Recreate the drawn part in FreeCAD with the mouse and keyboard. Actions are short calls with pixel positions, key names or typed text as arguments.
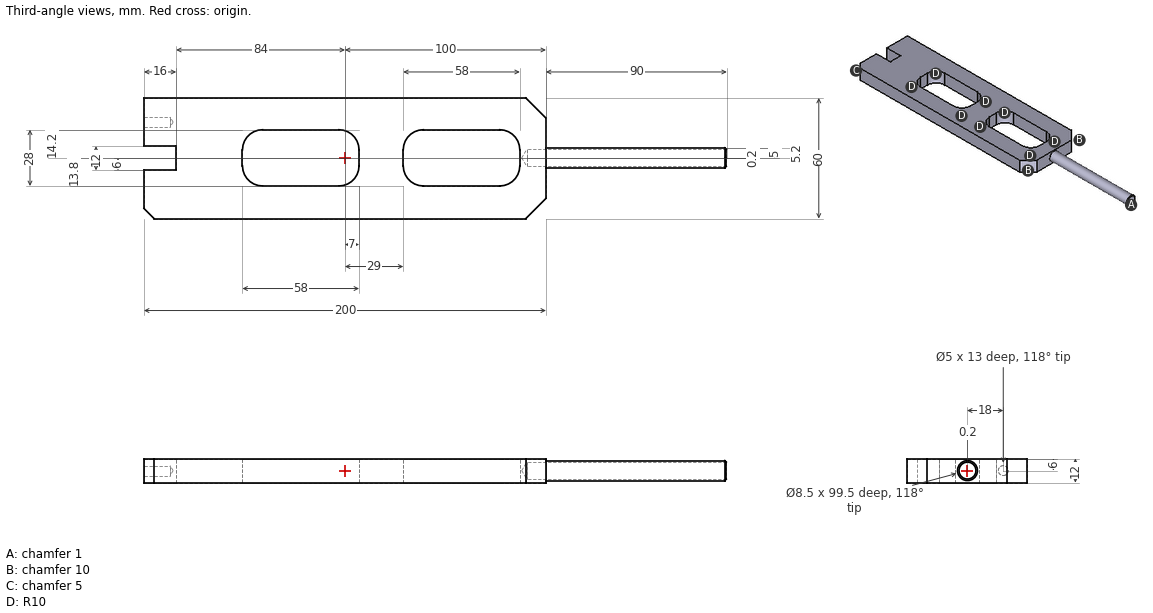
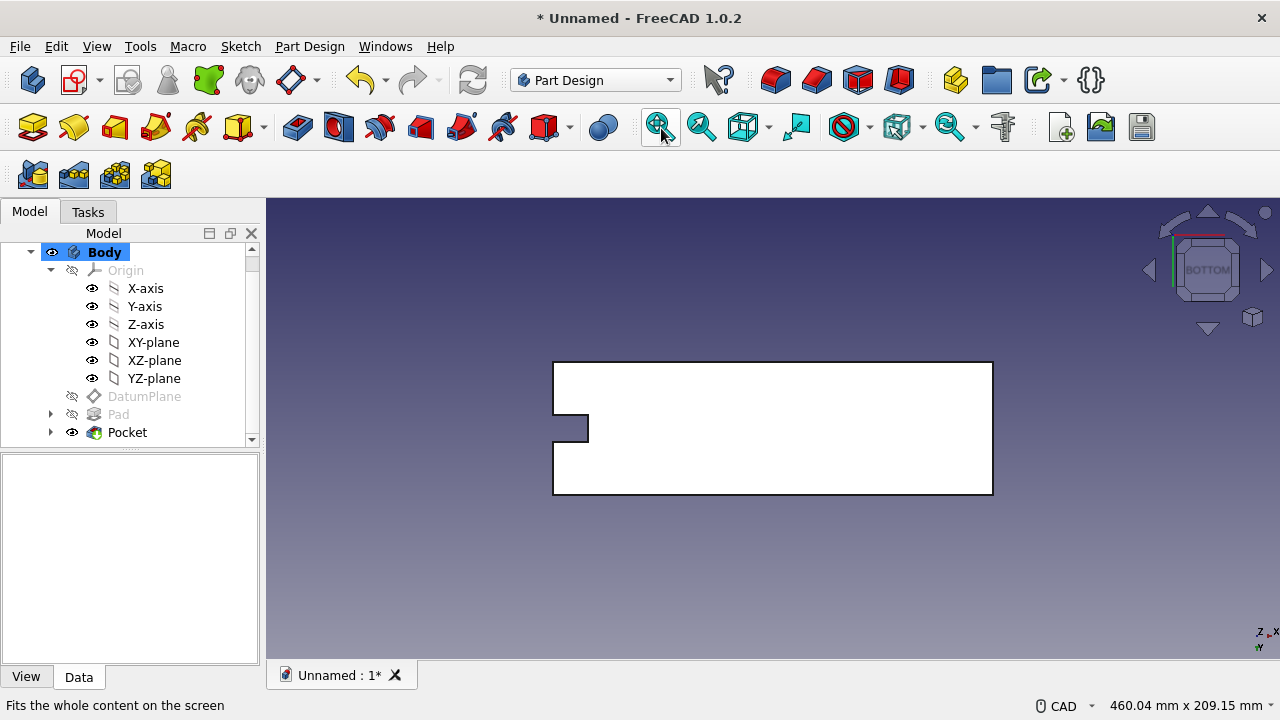
key(0)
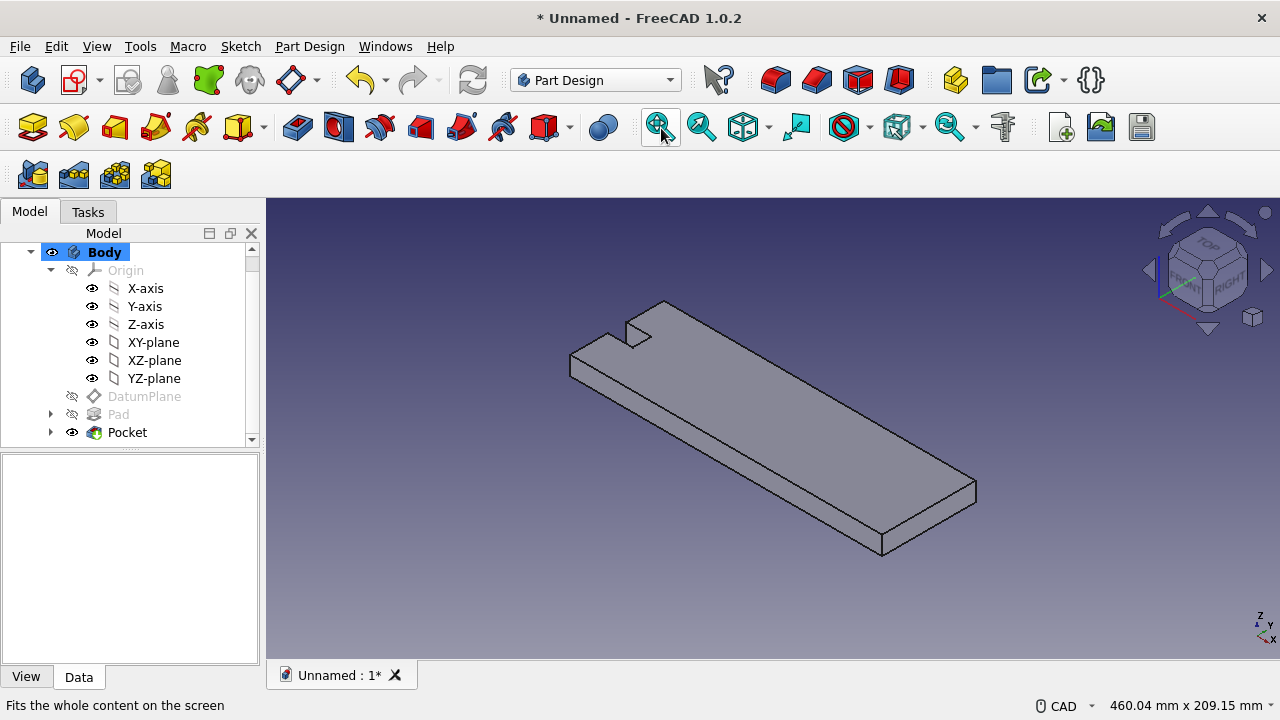
click(862, 468)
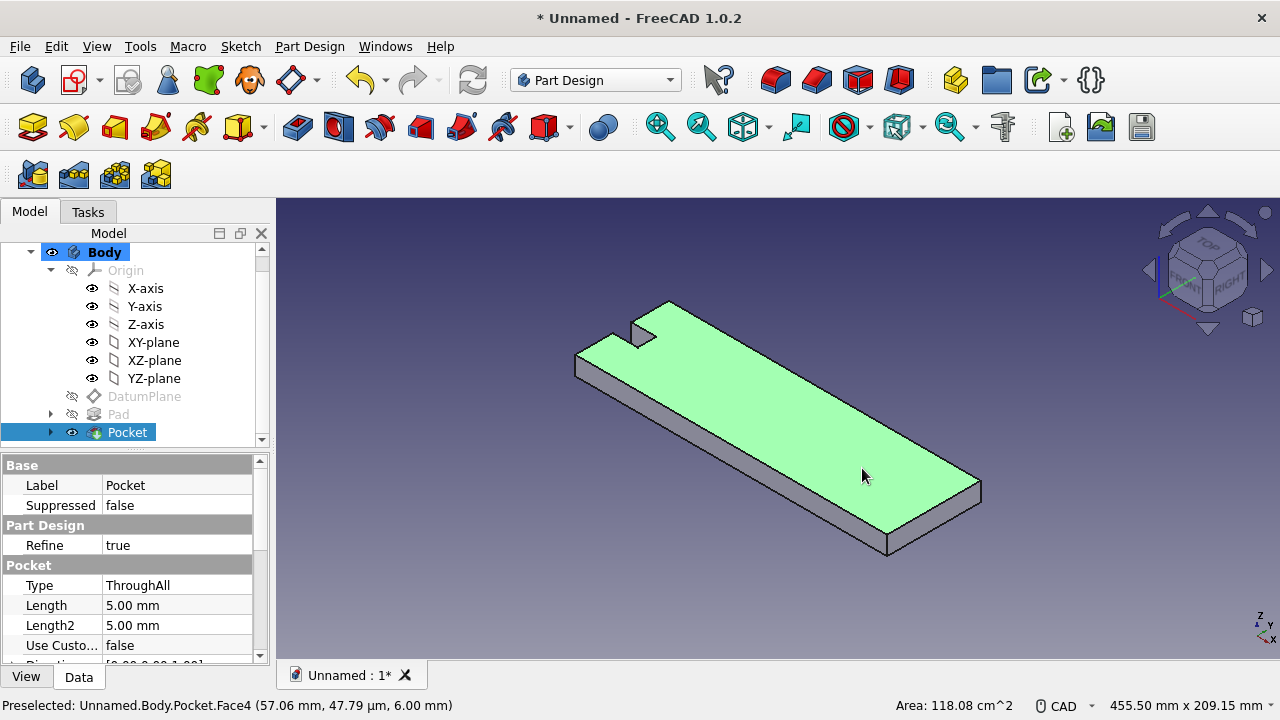
click(74, 80)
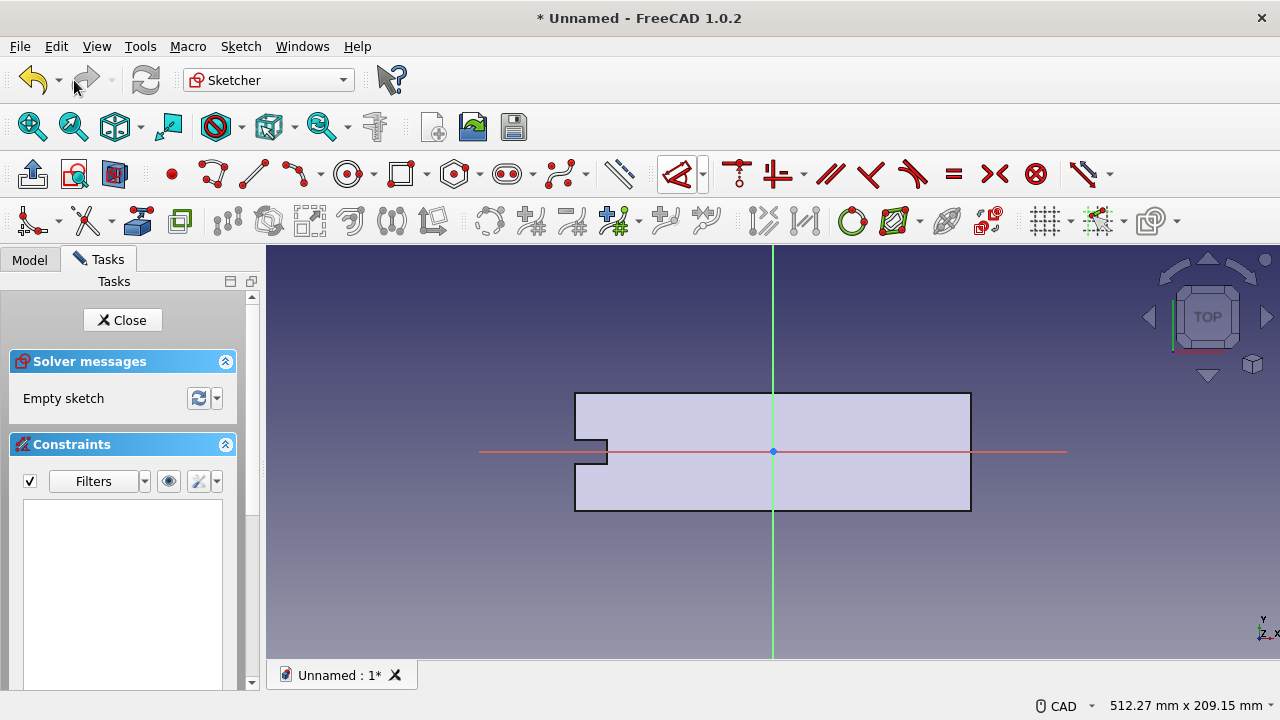
scroll(736, 452, up, 8)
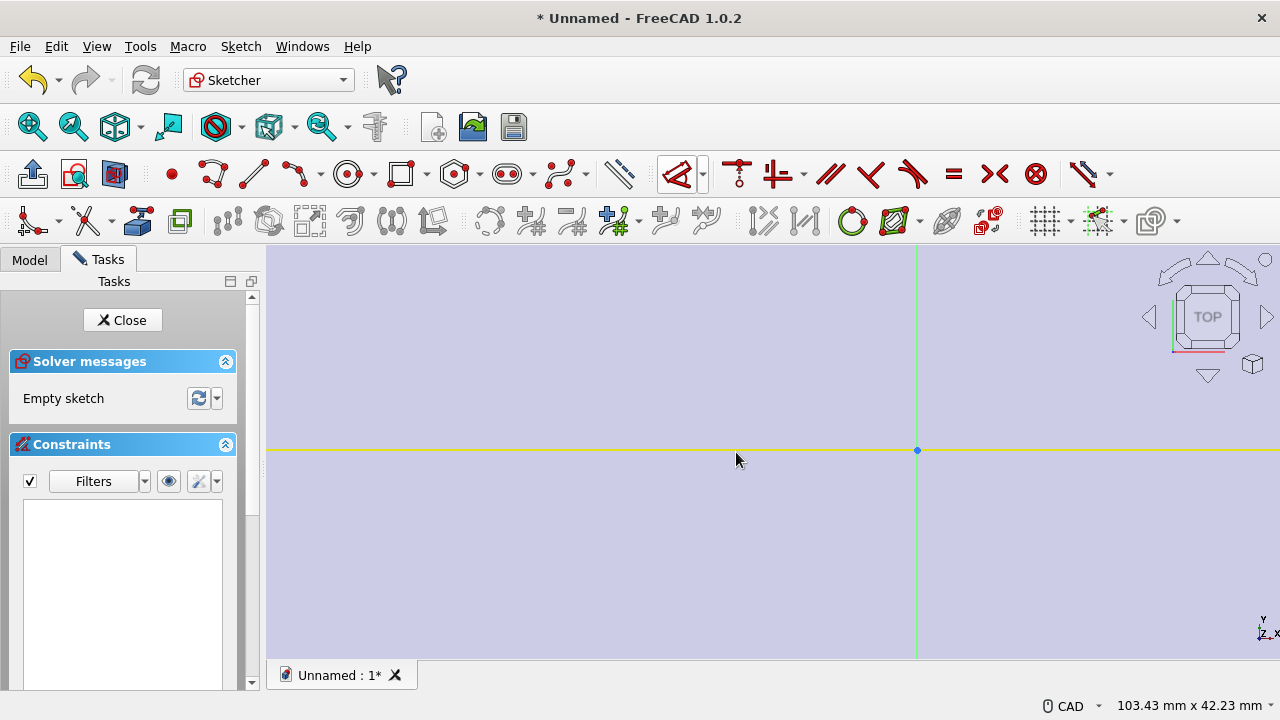
click(400, 174)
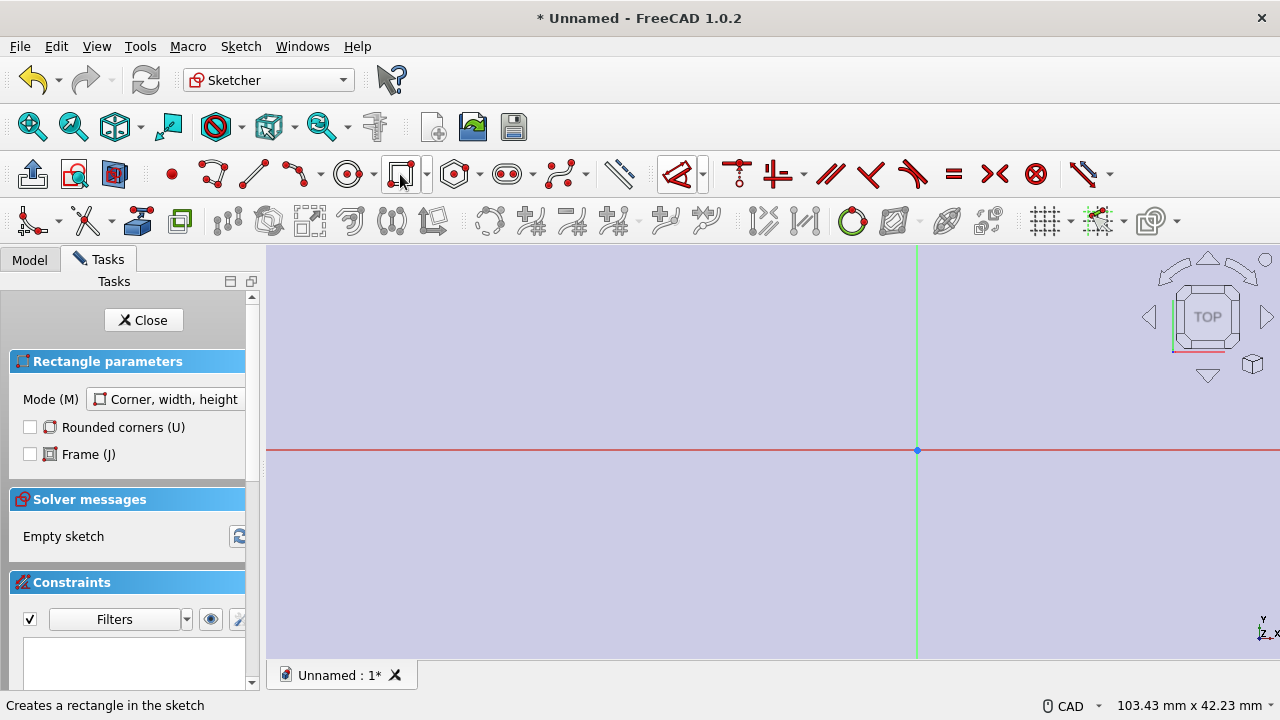
click(417, 311)
move(986, 585)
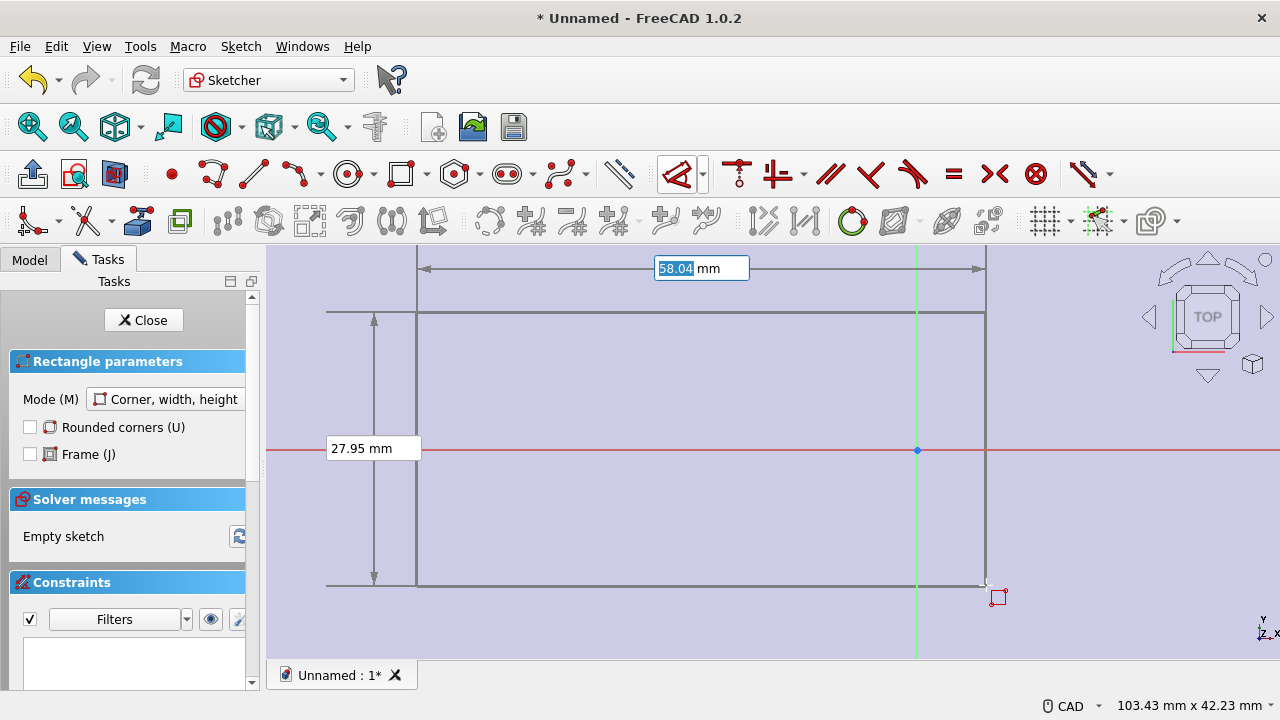
text(58)
key(Tab)
text(28)
key(Return)
key(Escape)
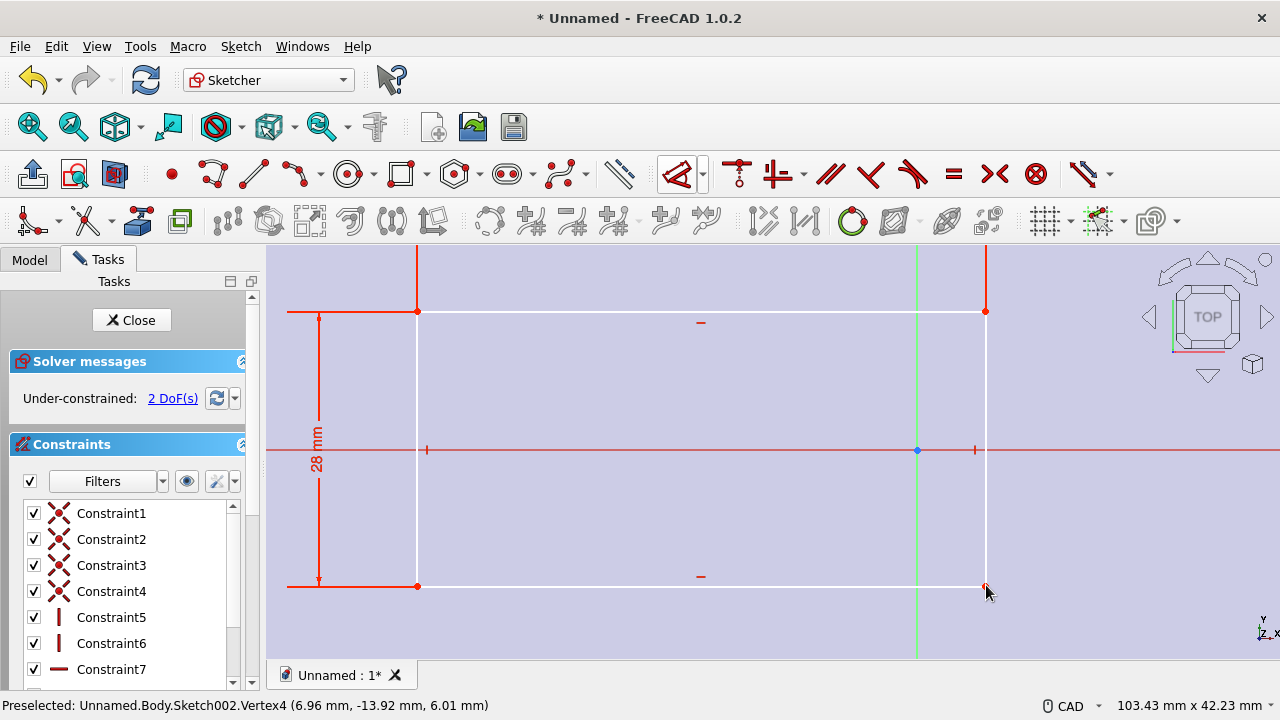
click(986, 587)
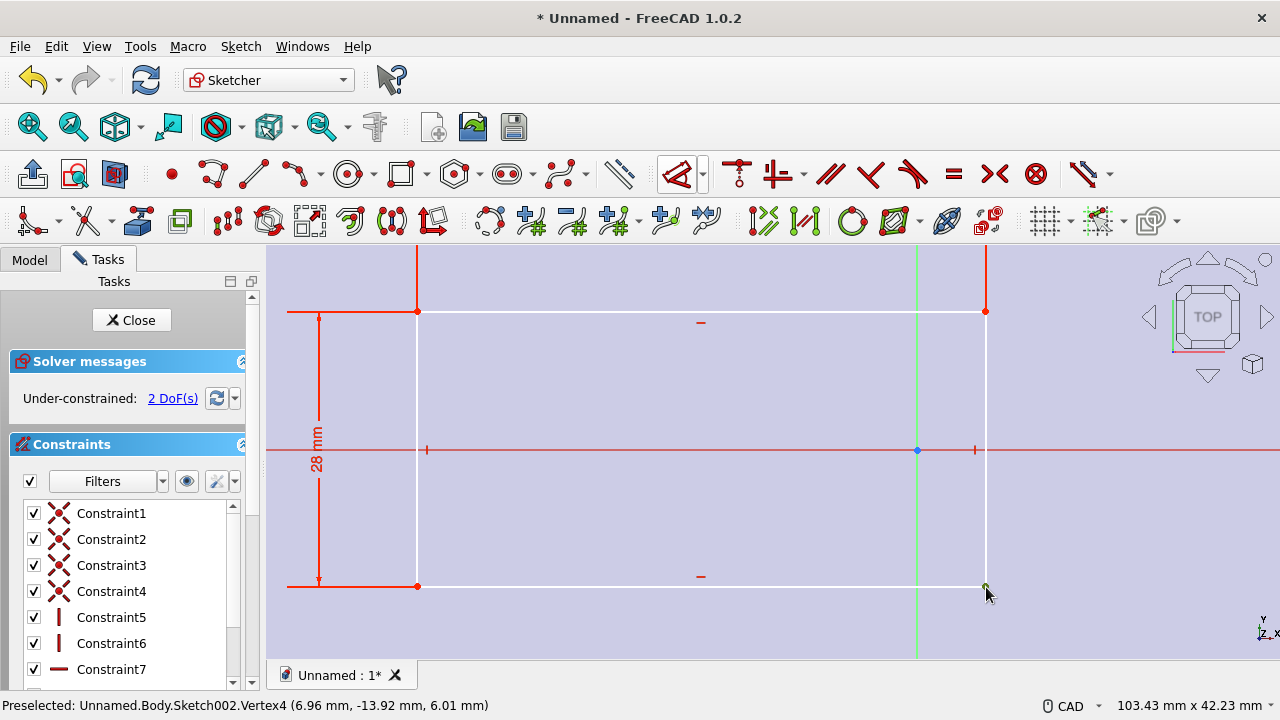
click(702, 174)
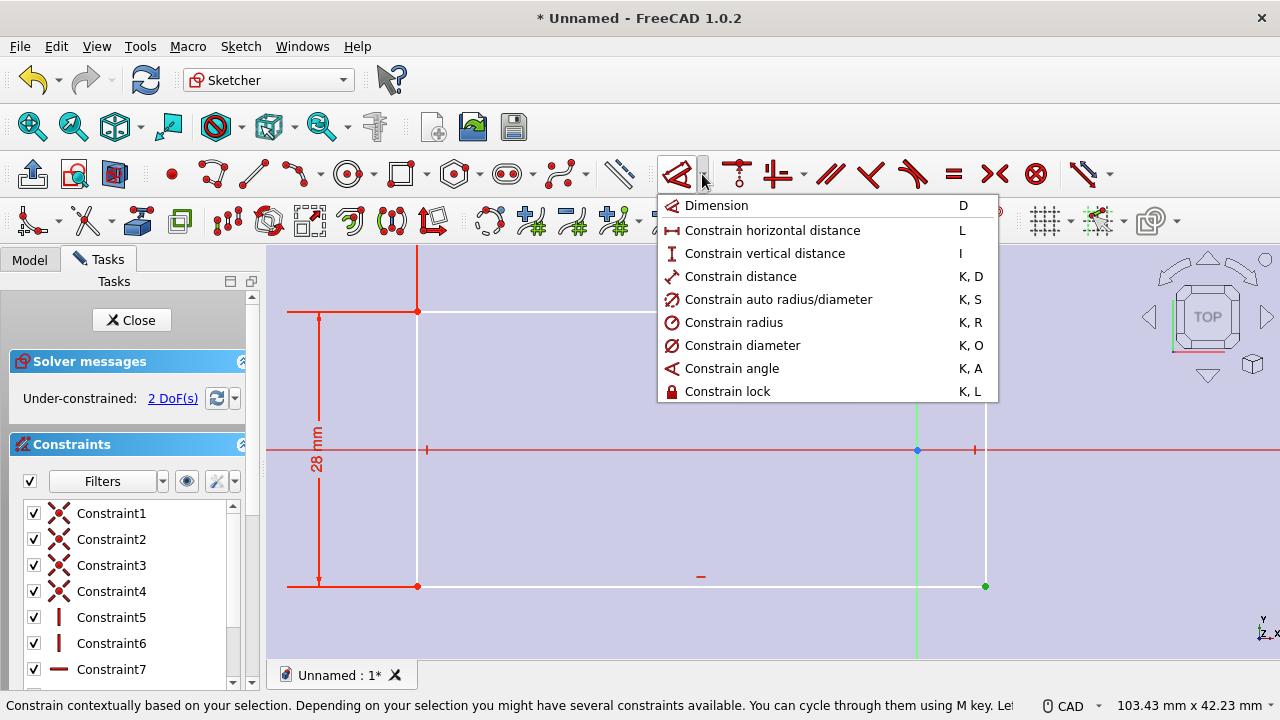
click(828, 230)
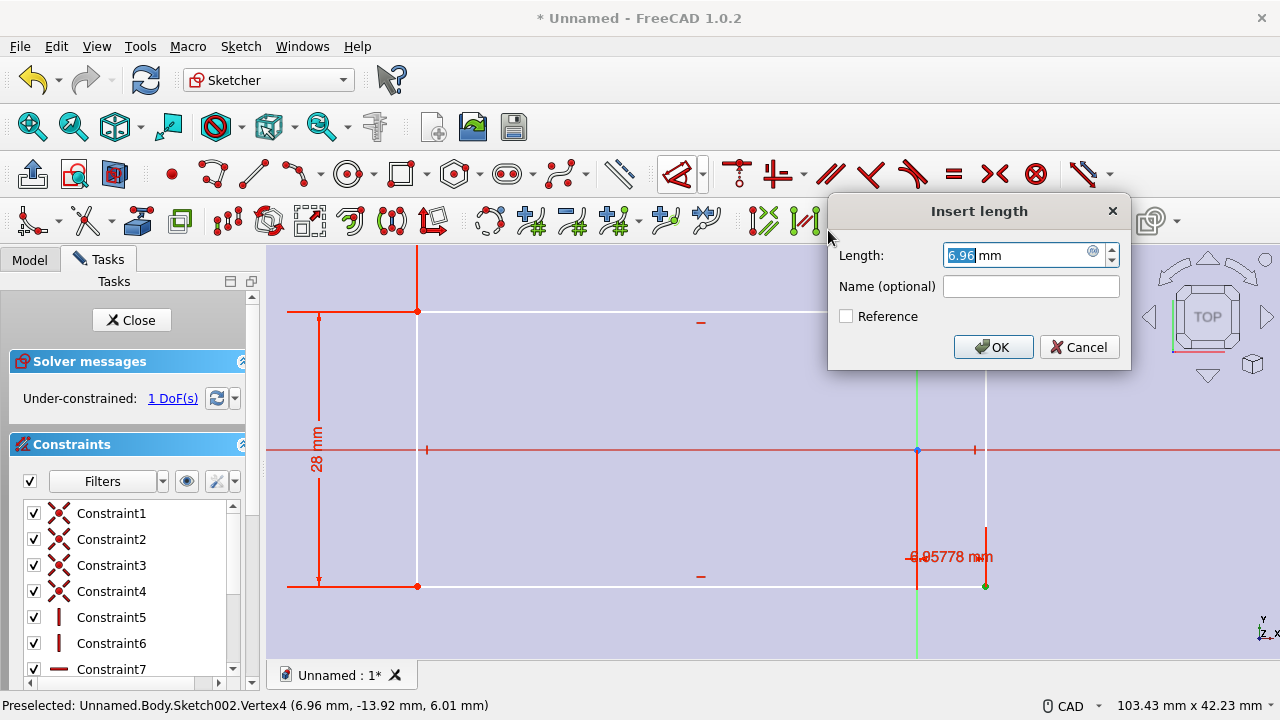
text(7)
key(Return)